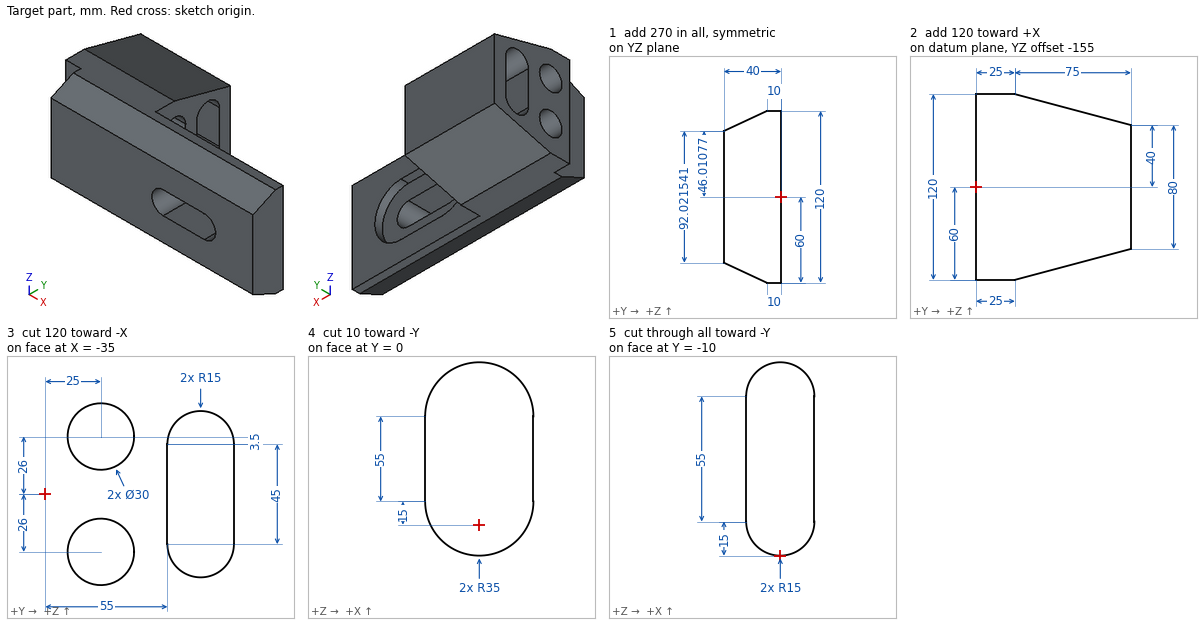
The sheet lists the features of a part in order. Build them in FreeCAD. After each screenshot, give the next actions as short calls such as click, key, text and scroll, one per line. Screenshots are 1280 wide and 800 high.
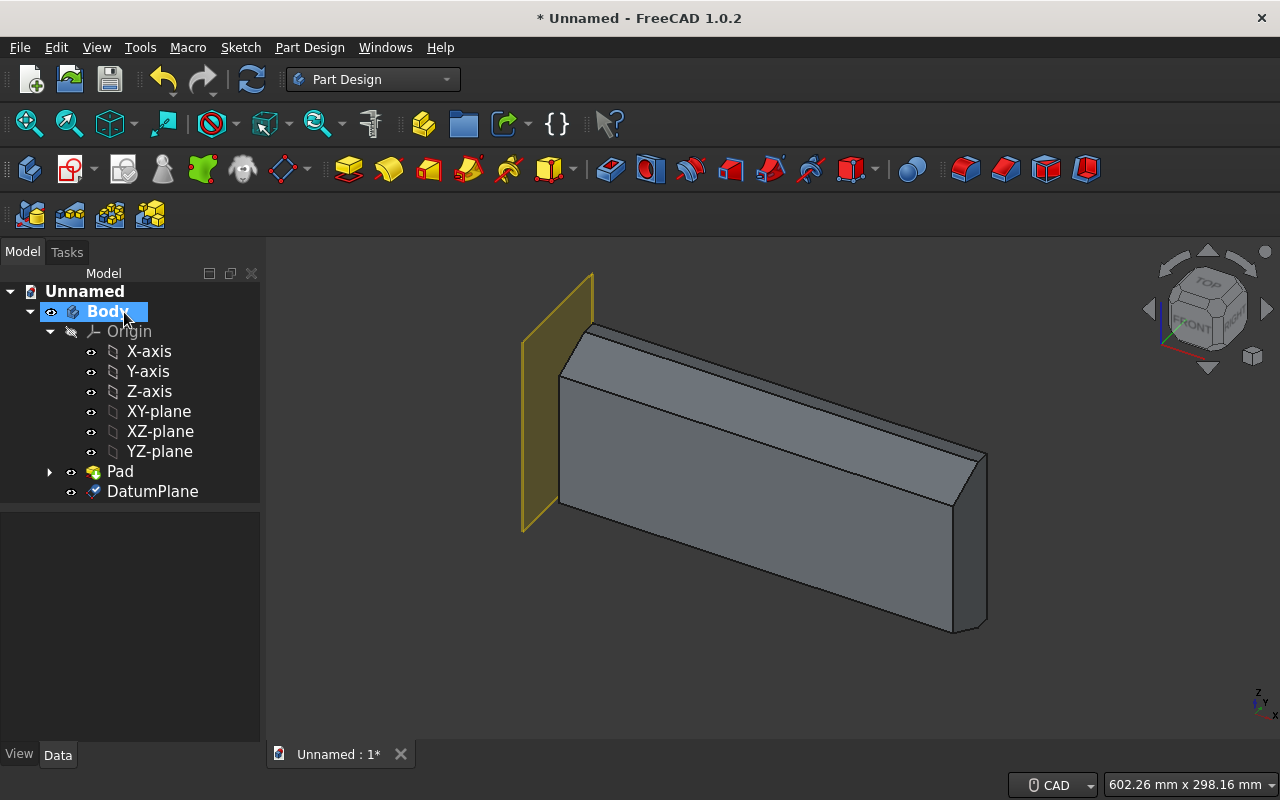
click(116, 492)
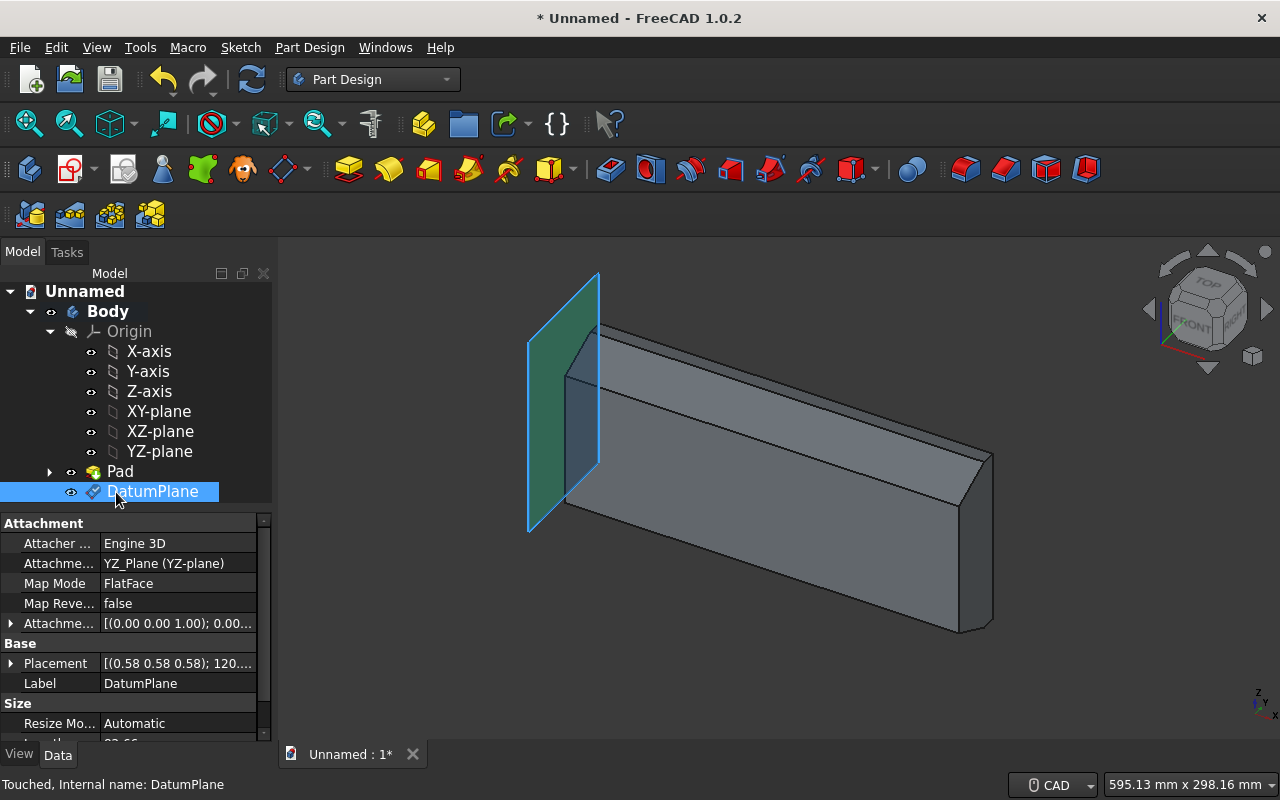
click(70, 170)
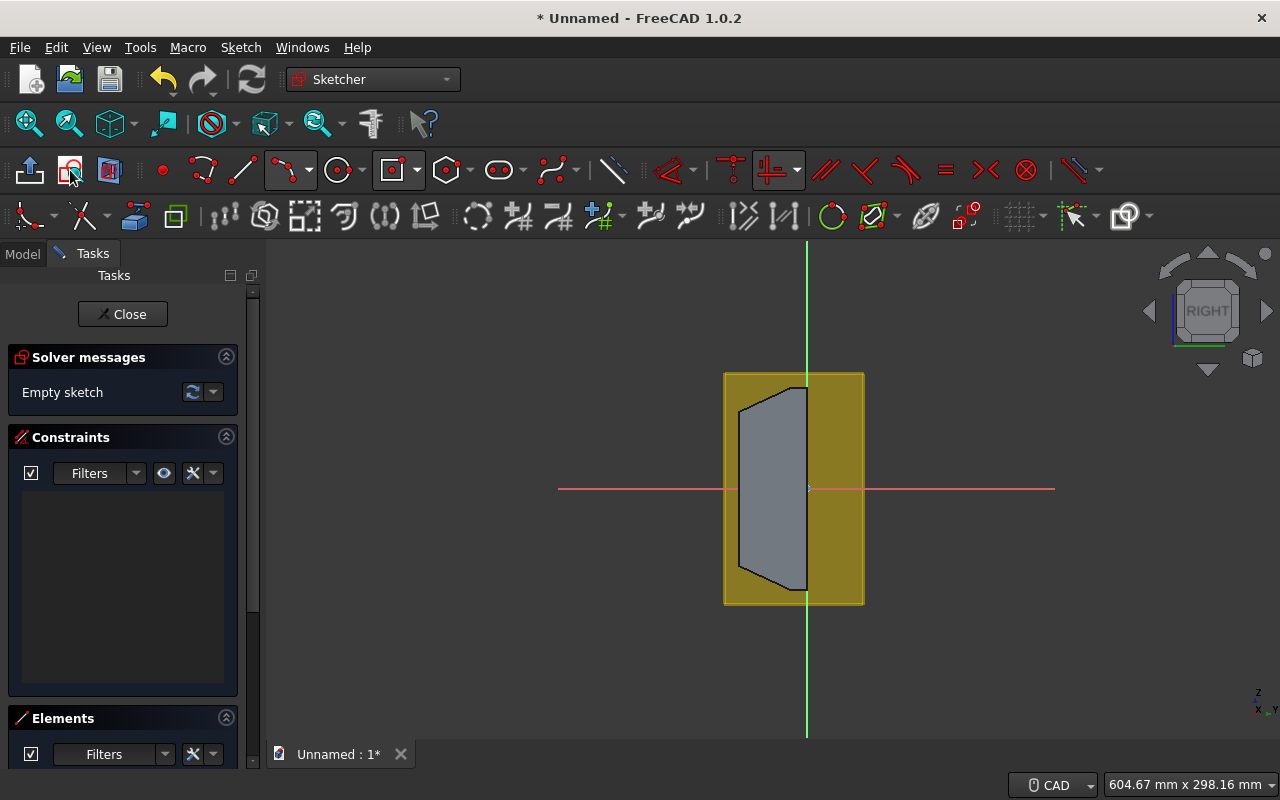
click(110, 170)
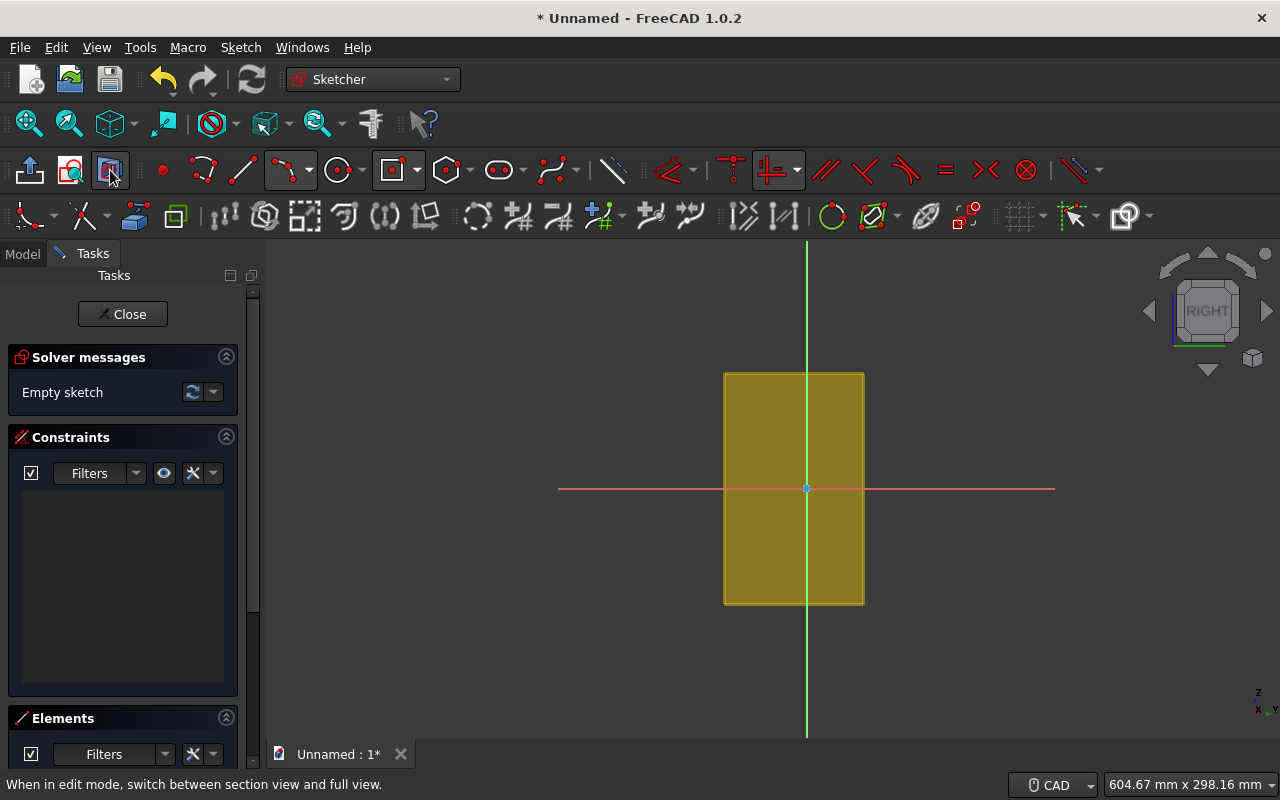
scroll(1115, 489, up, 2)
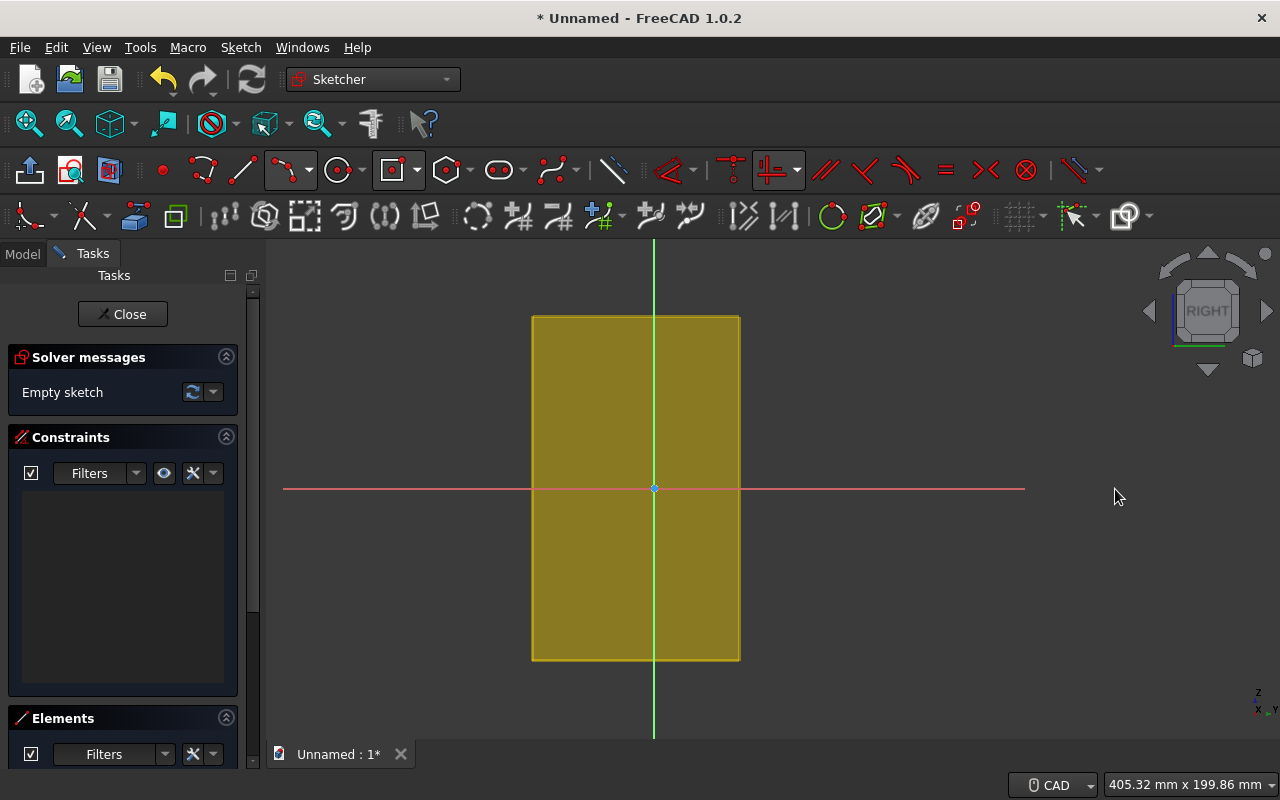
click(204, 170)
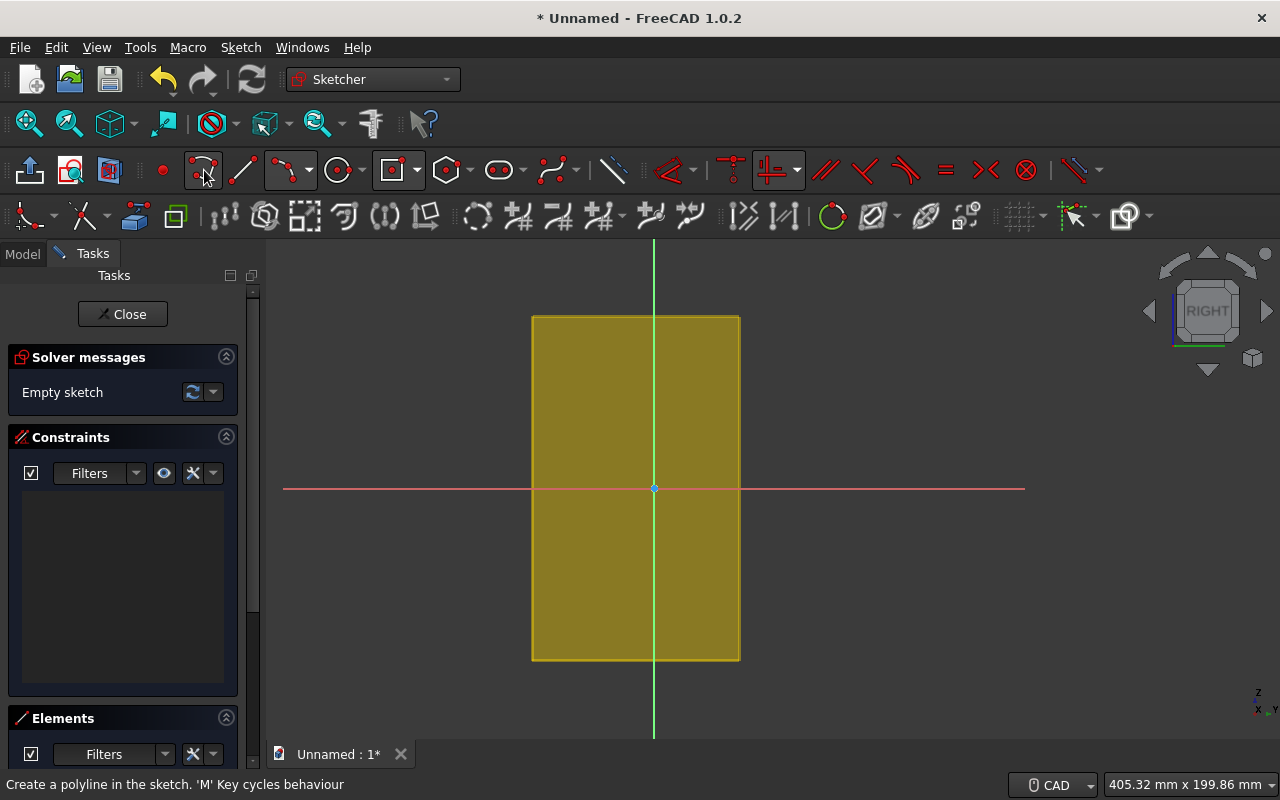
click(654, 639)
click(663, 339)
click(717, 339)
click(905, 389)
click(905, 589)
click(717, 639)
click(654, 640)
key(Escape)
key(Escape)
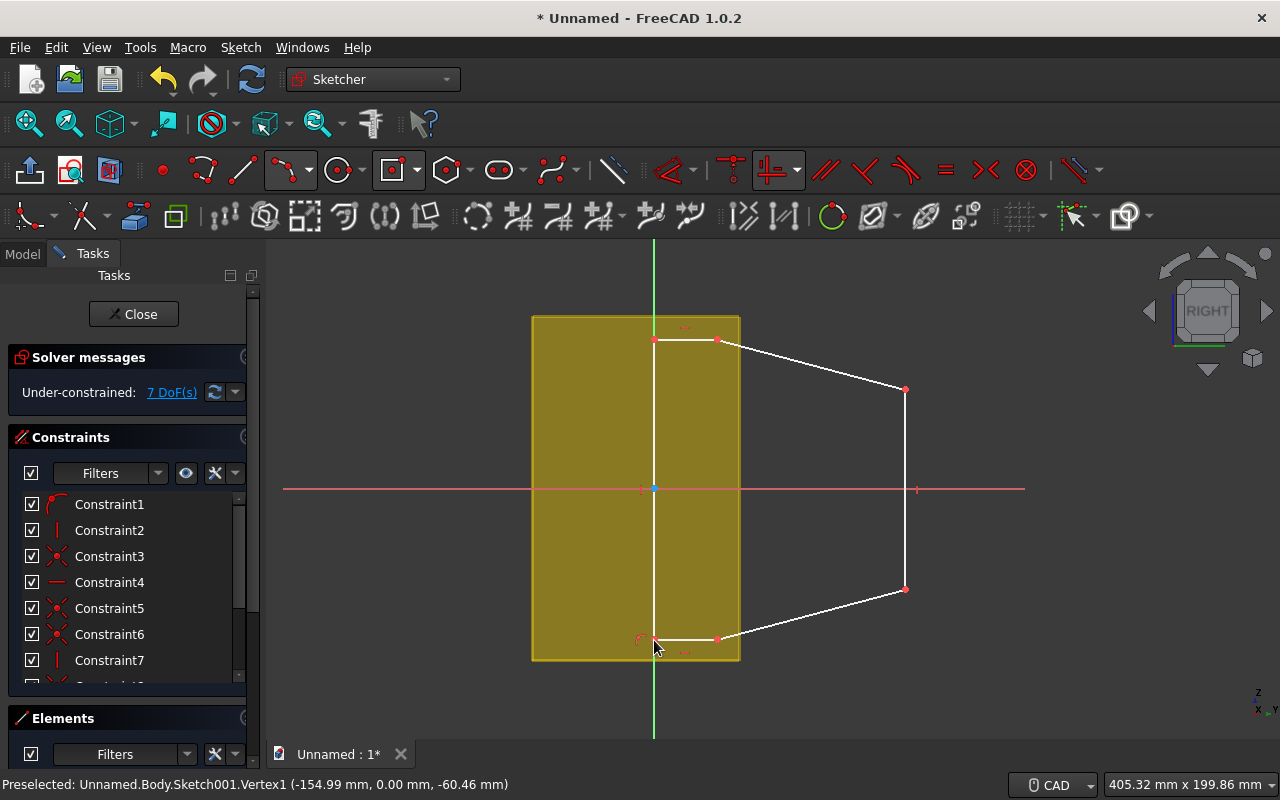
click(668, 170)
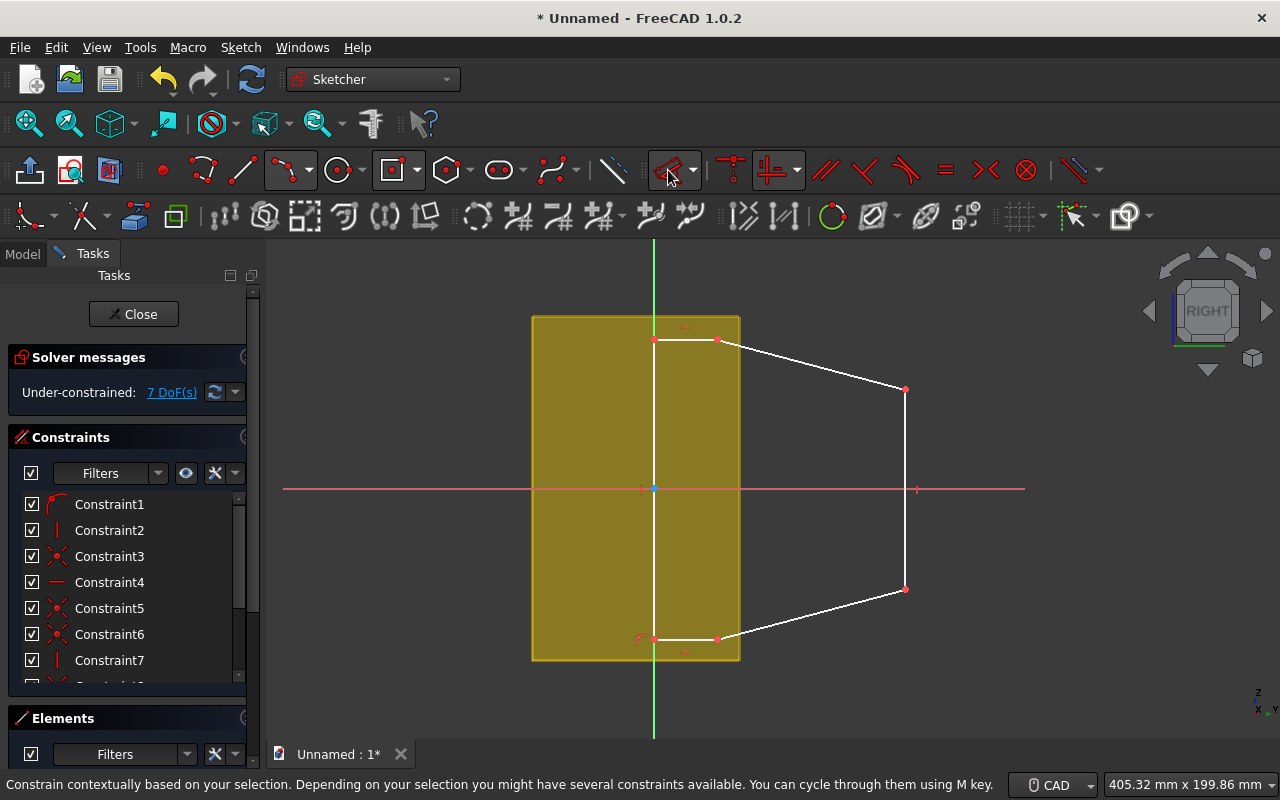
click(673, 340)
click(686, 306)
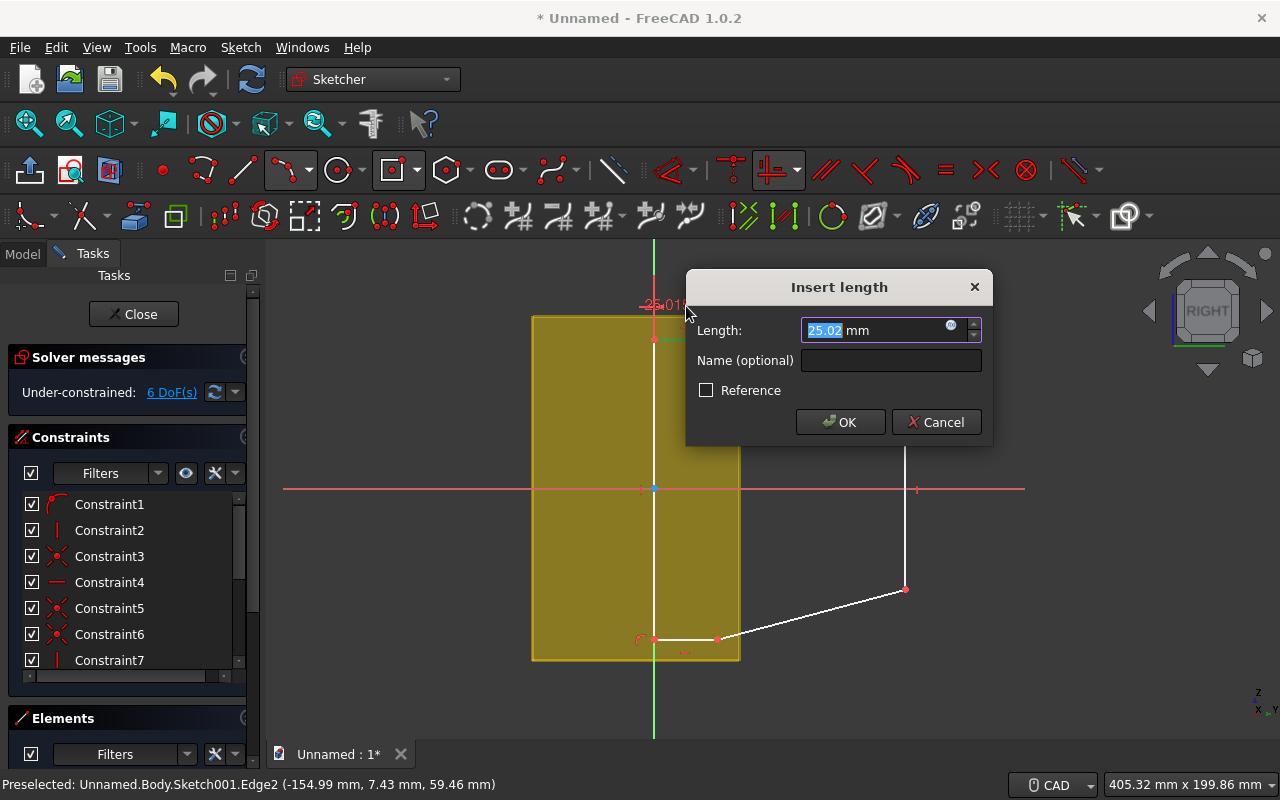
text(25)
key(Return)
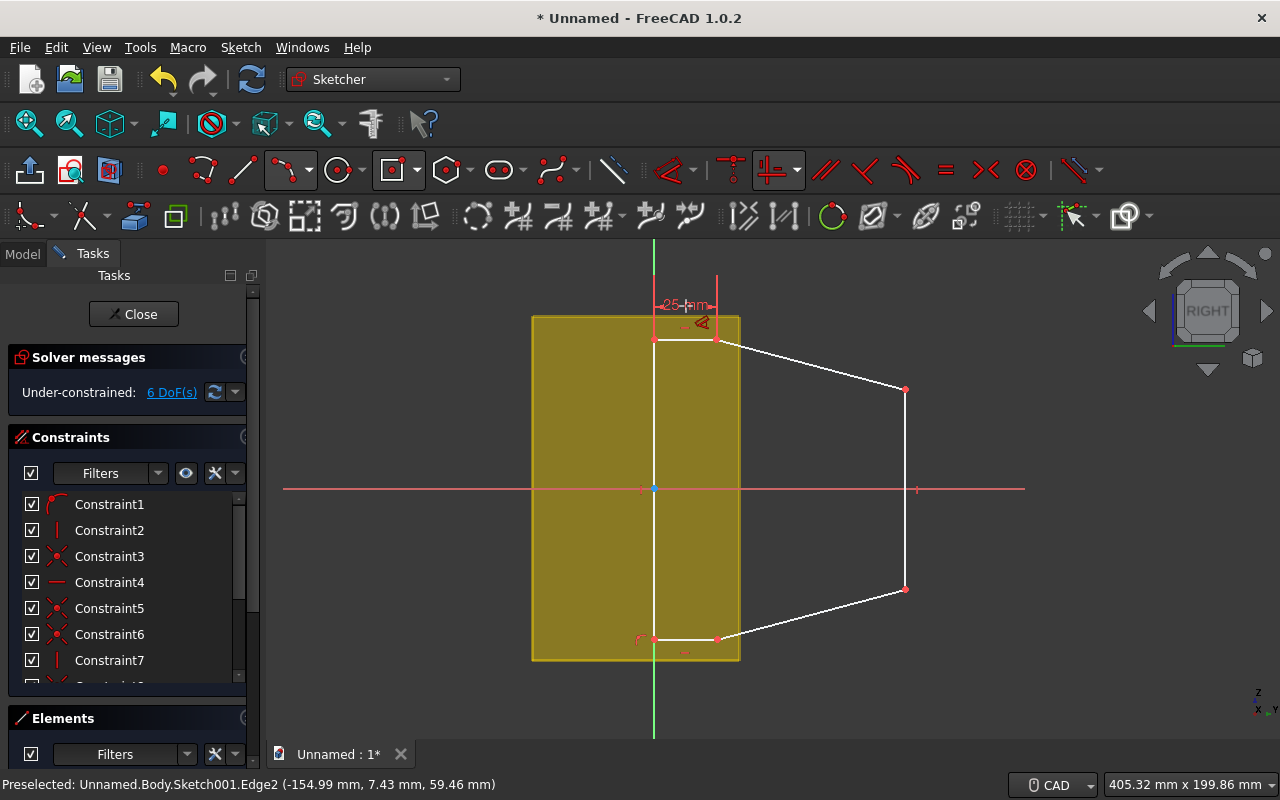
click(905, 450)
click(939, 444)